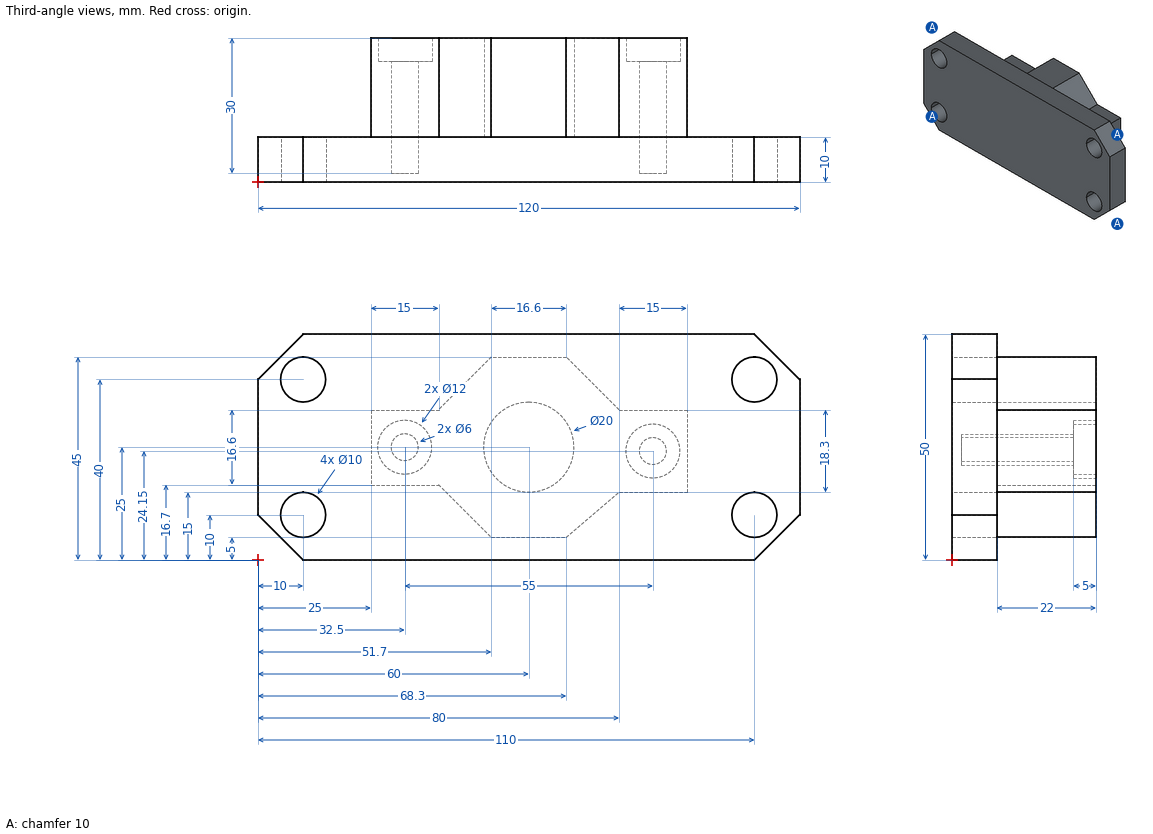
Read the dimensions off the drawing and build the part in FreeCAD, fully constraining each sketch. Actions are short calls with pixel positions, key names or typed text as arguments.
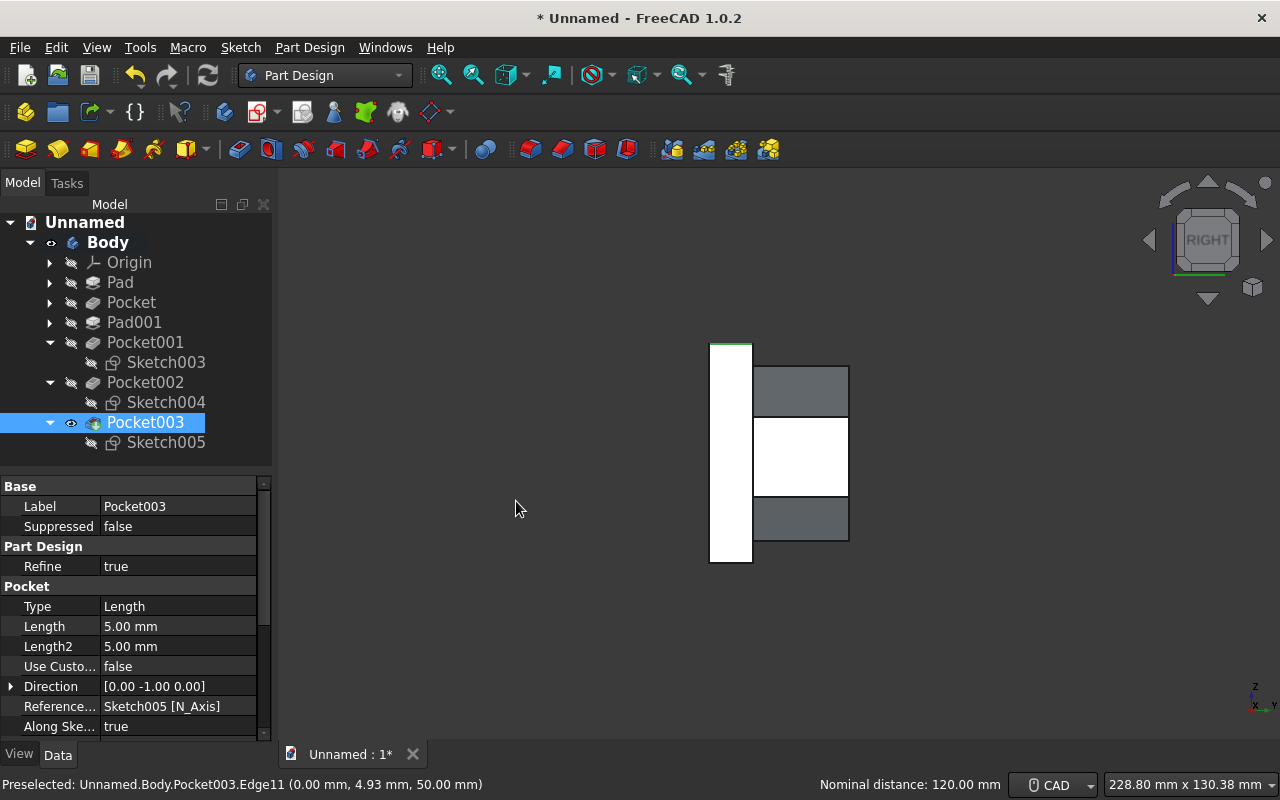
click(442, 76)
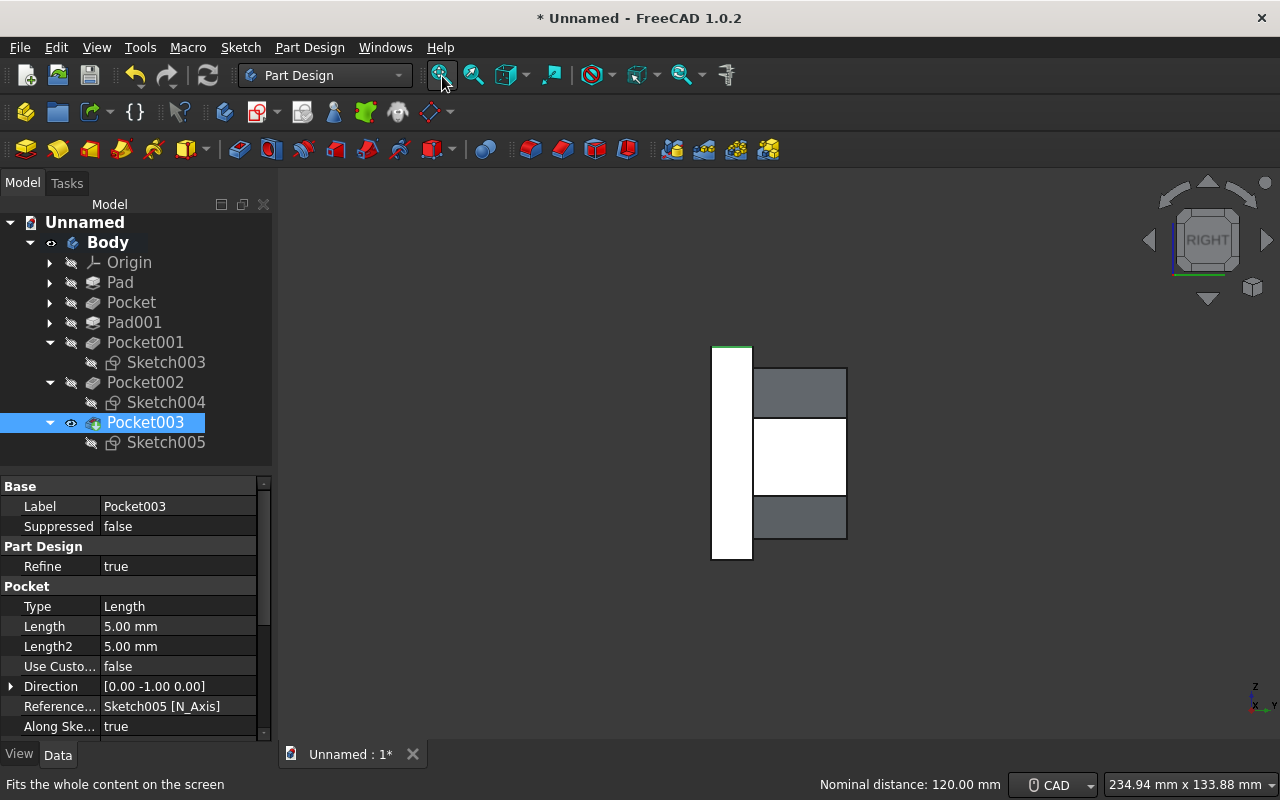
click(732, 559, ctrl)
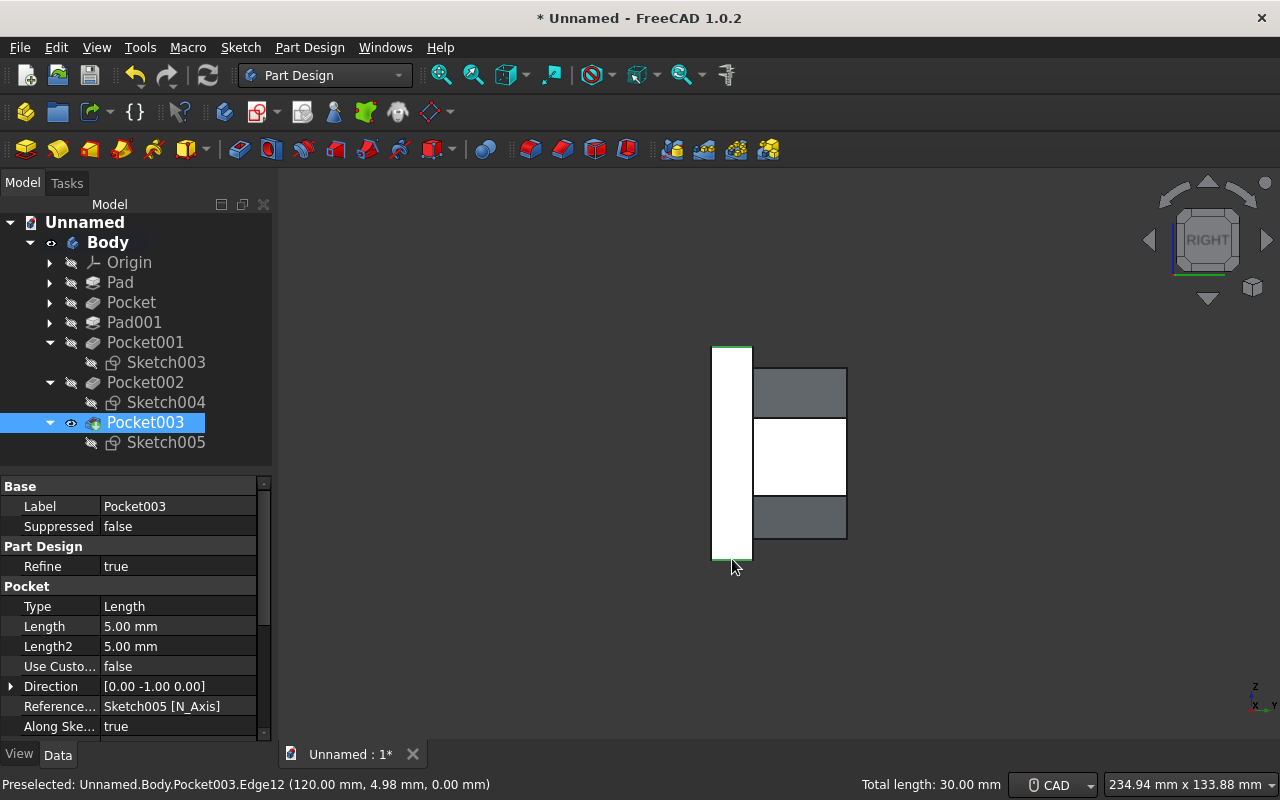
key(5)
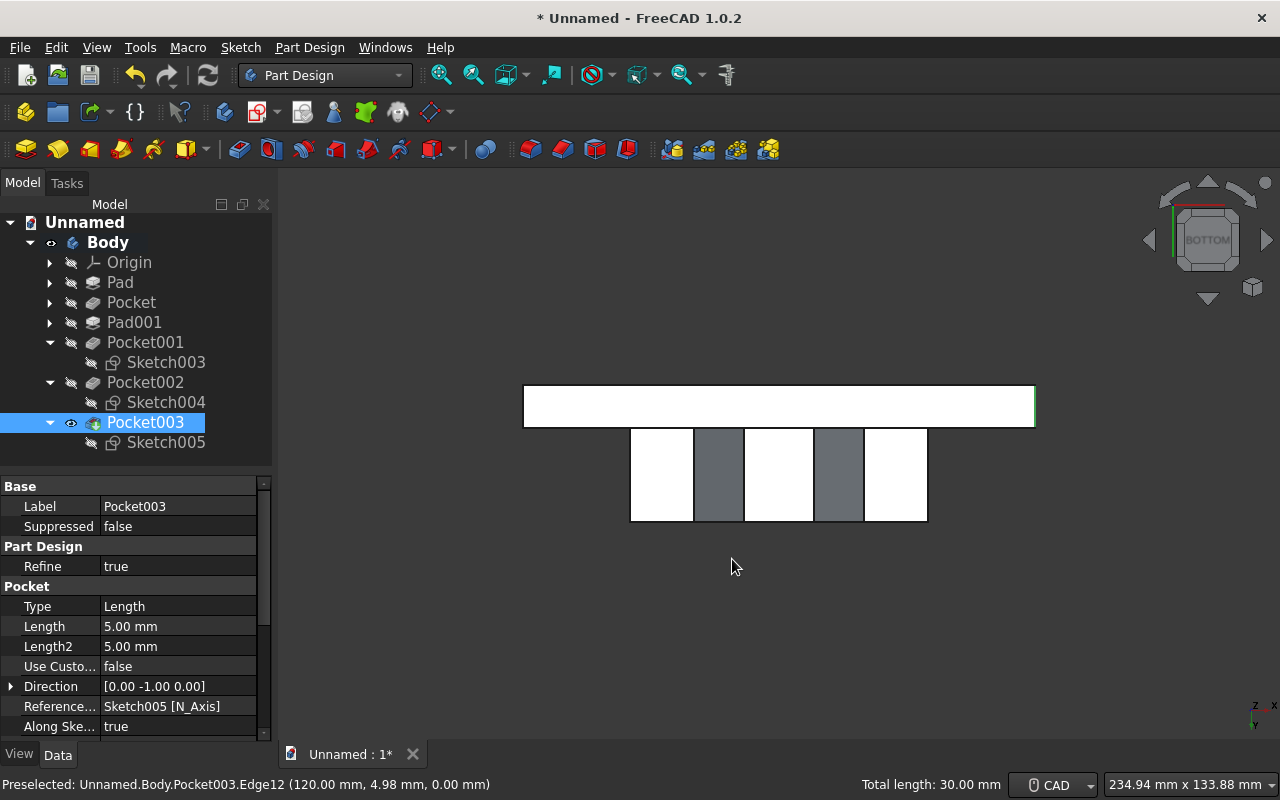
click(523, 406, ctrl)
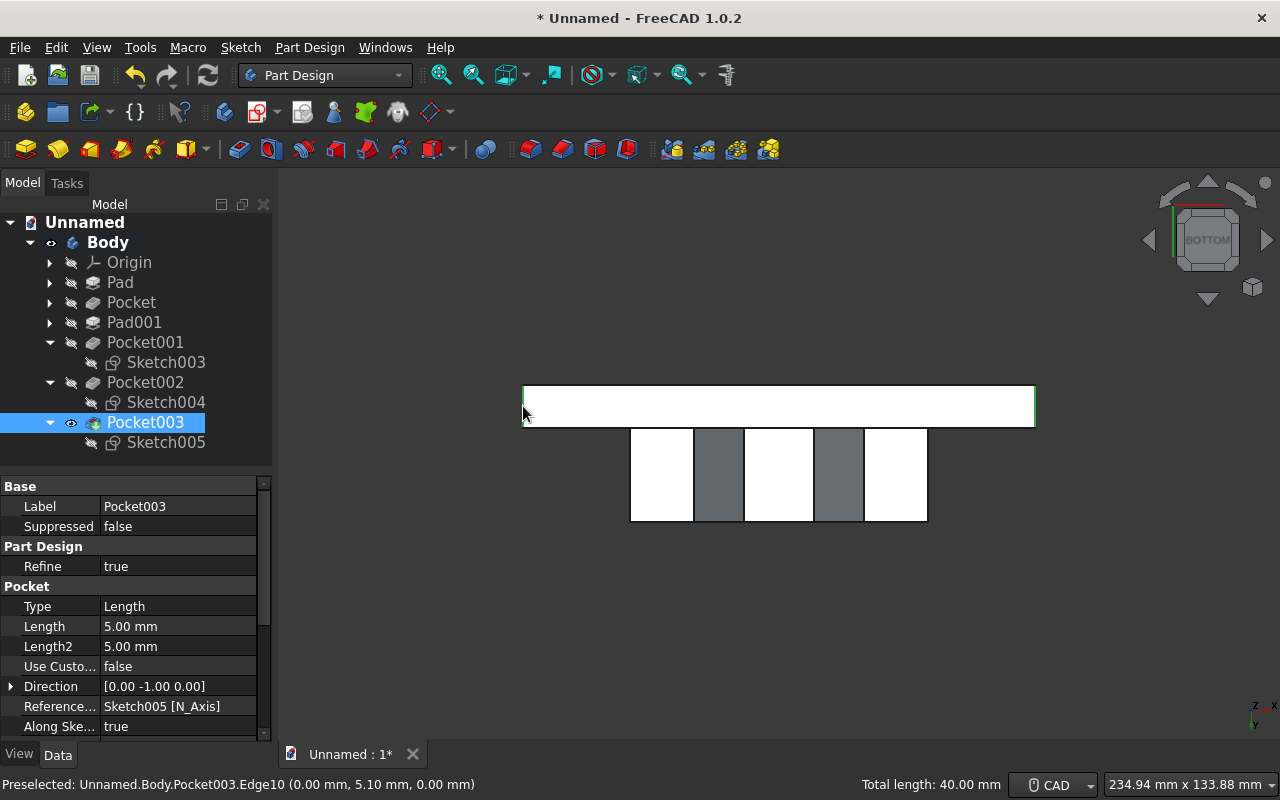
click(564, 150)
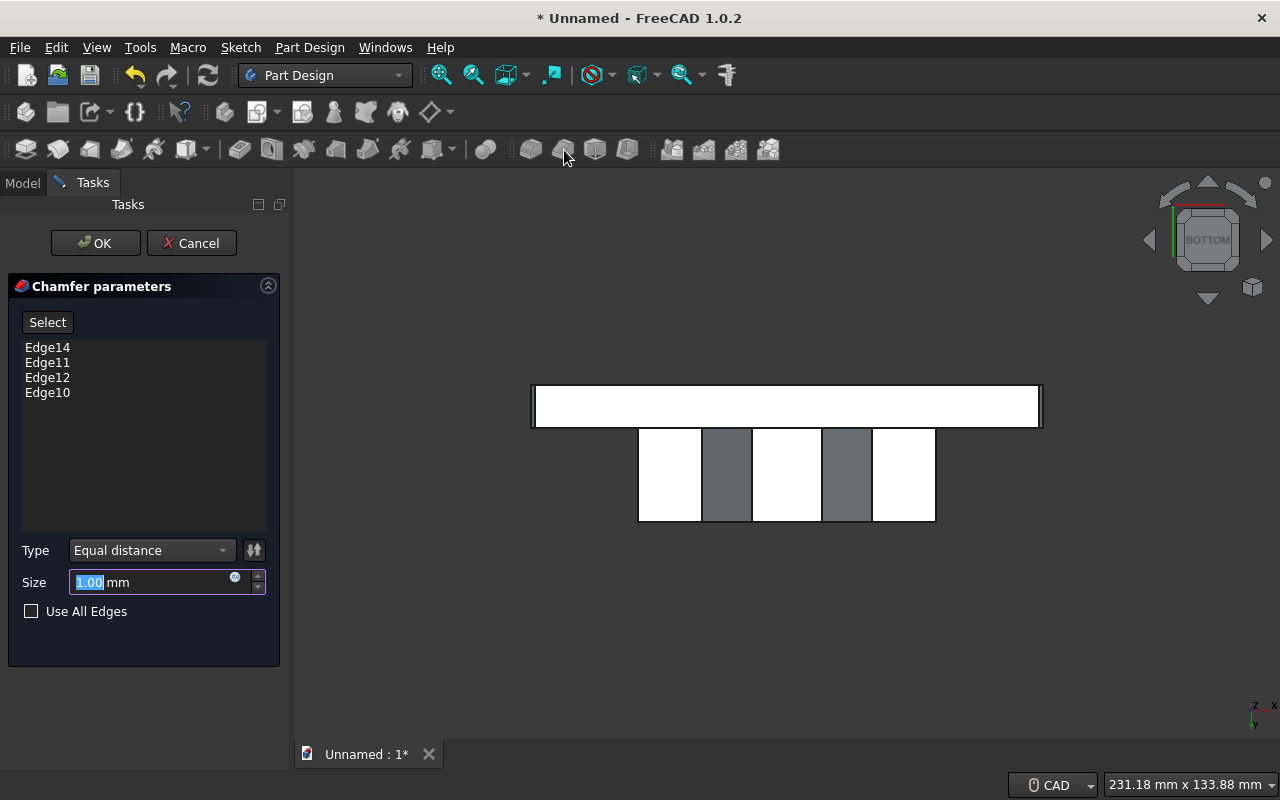
text(10)
key(Tab)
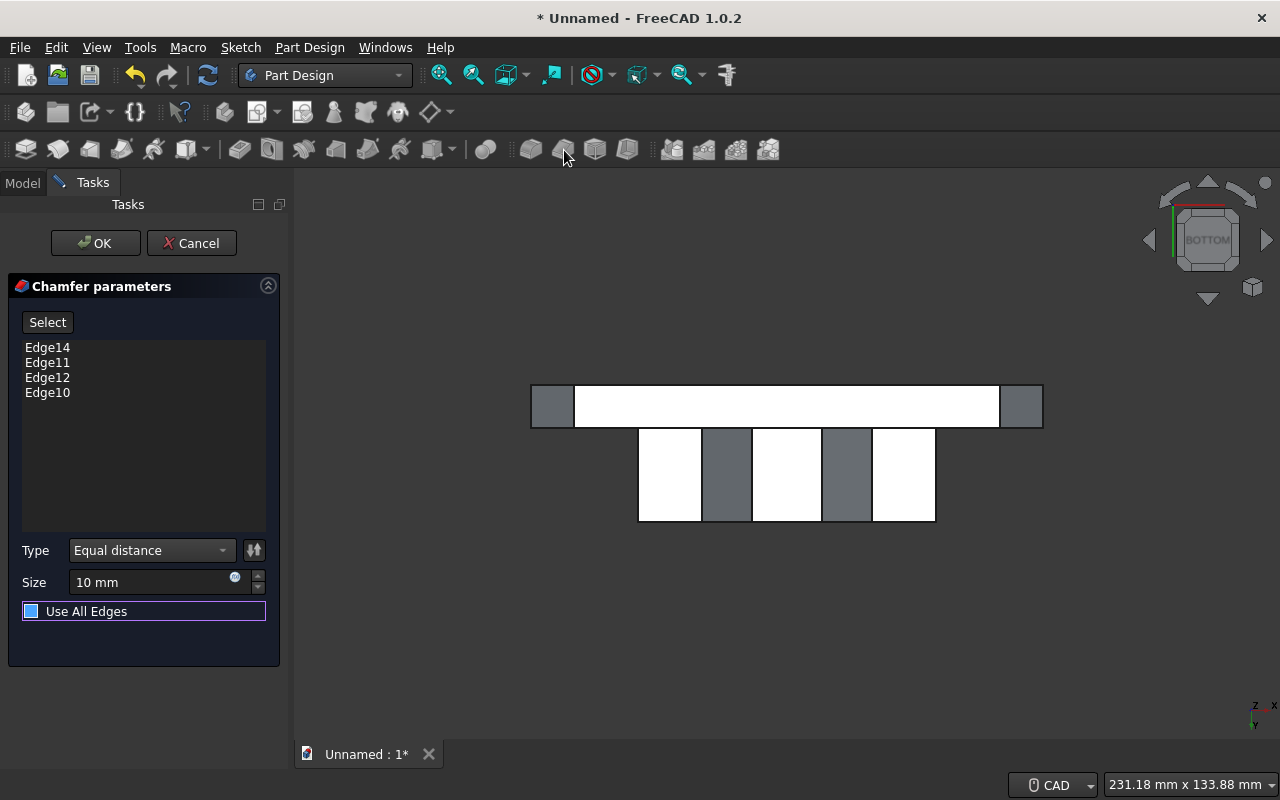
click(96, 243)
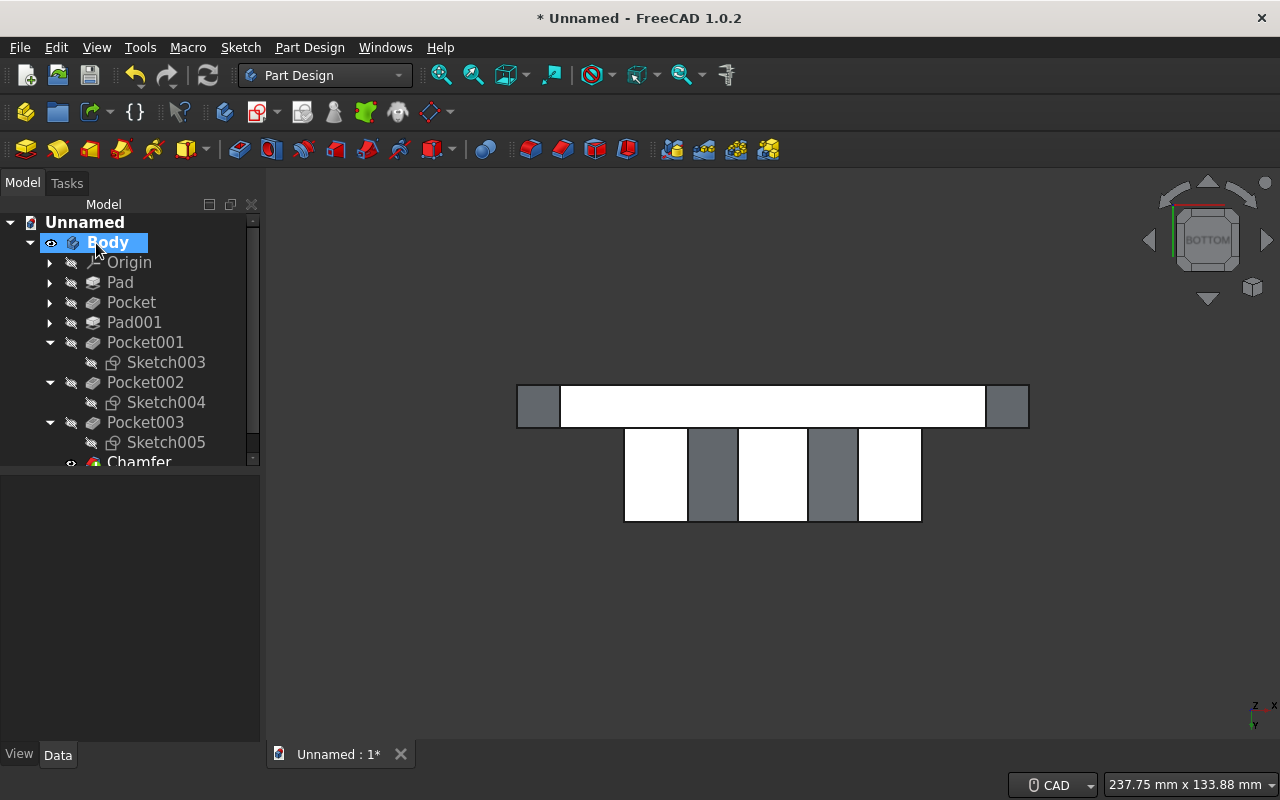
key(0)